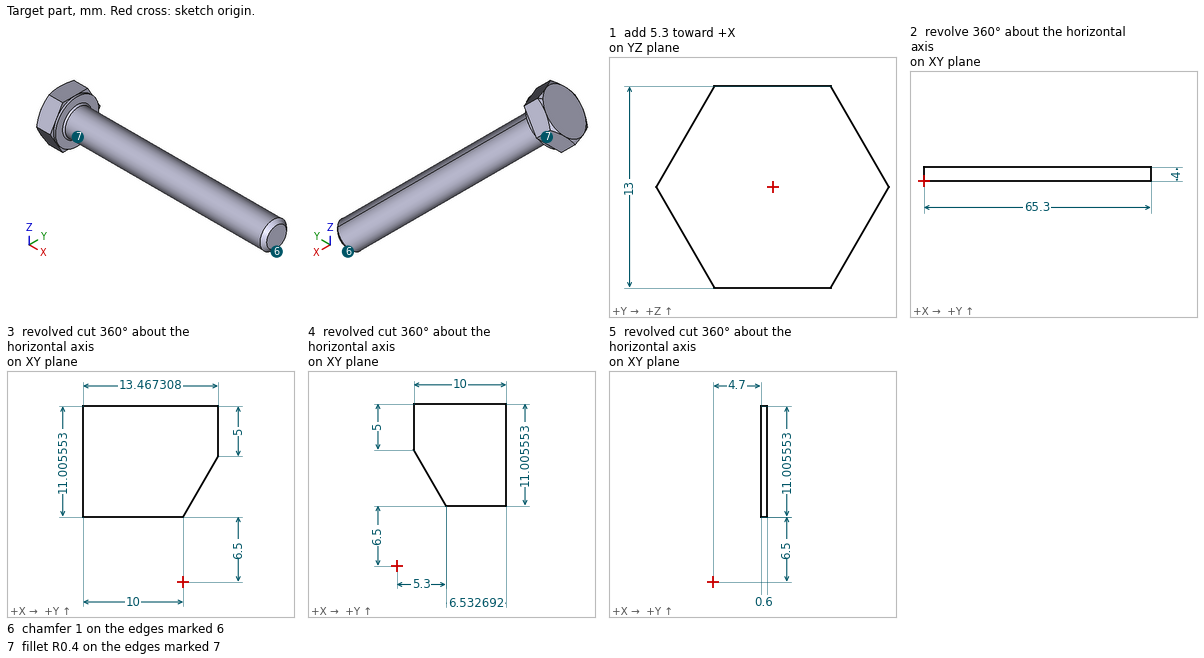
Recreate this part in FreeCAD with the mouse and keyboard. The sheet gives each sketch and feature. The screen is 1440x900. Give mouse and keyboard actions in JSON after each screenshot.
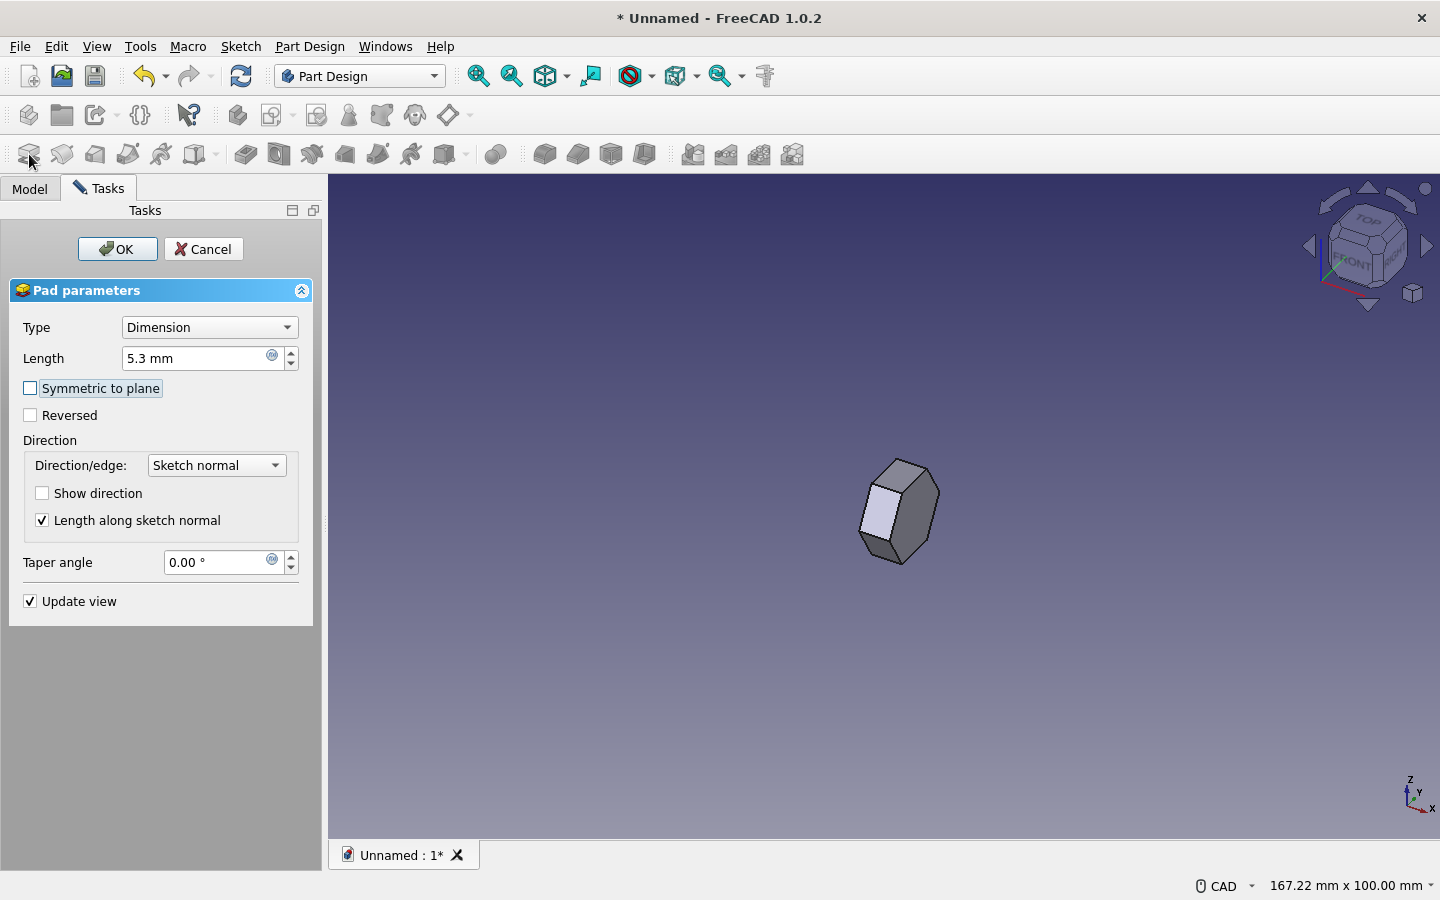
{"action": "left_click", "coordinate": [118, 249]}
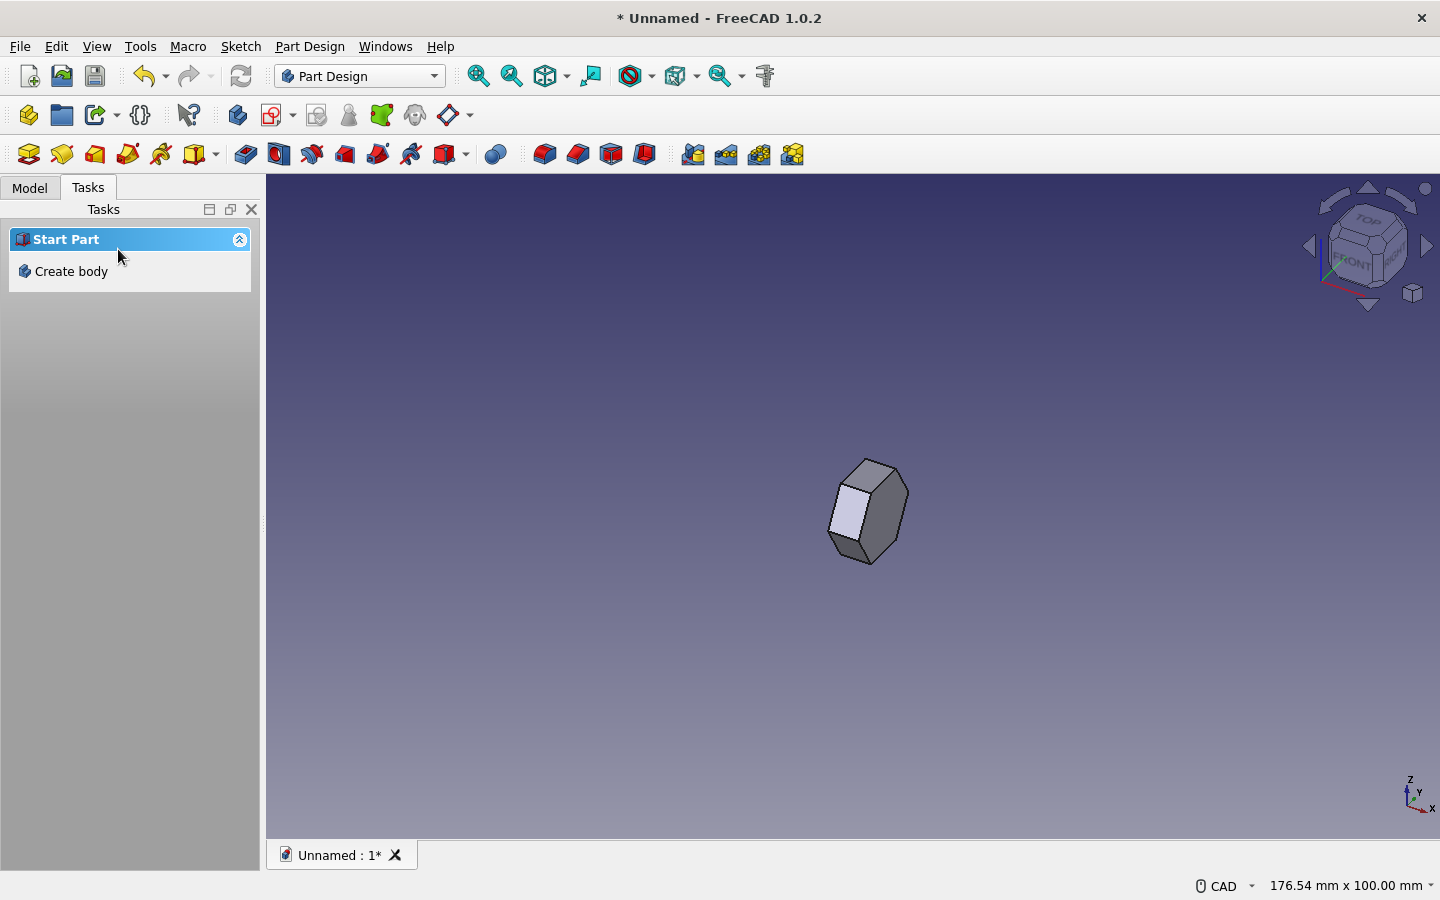
{"action": "left_click", "coordinate": [479, 76]}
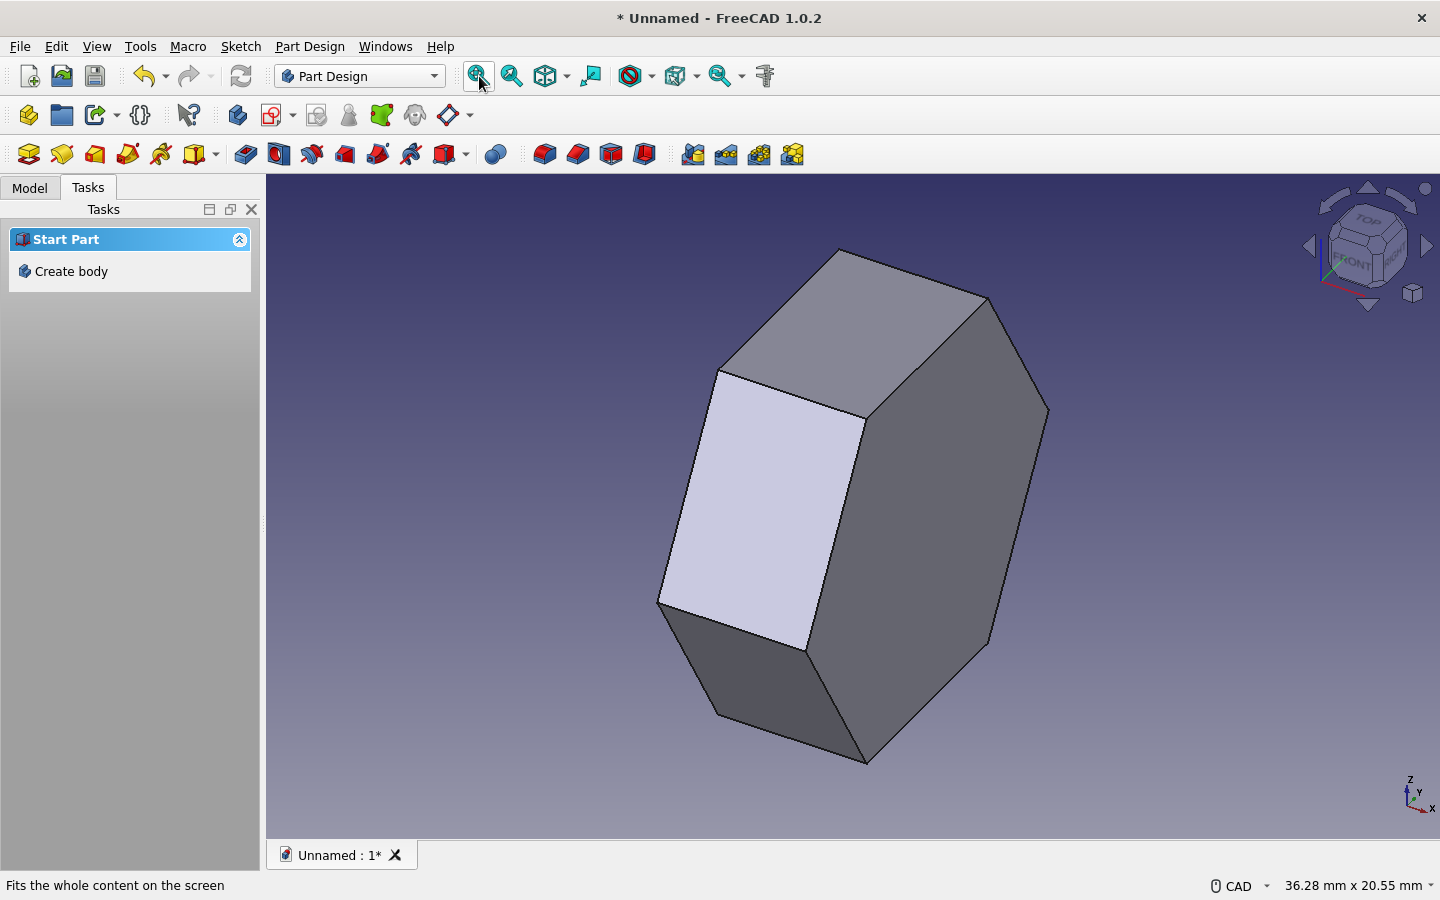
{"action": "left_click", "coordinate": [270, 116]}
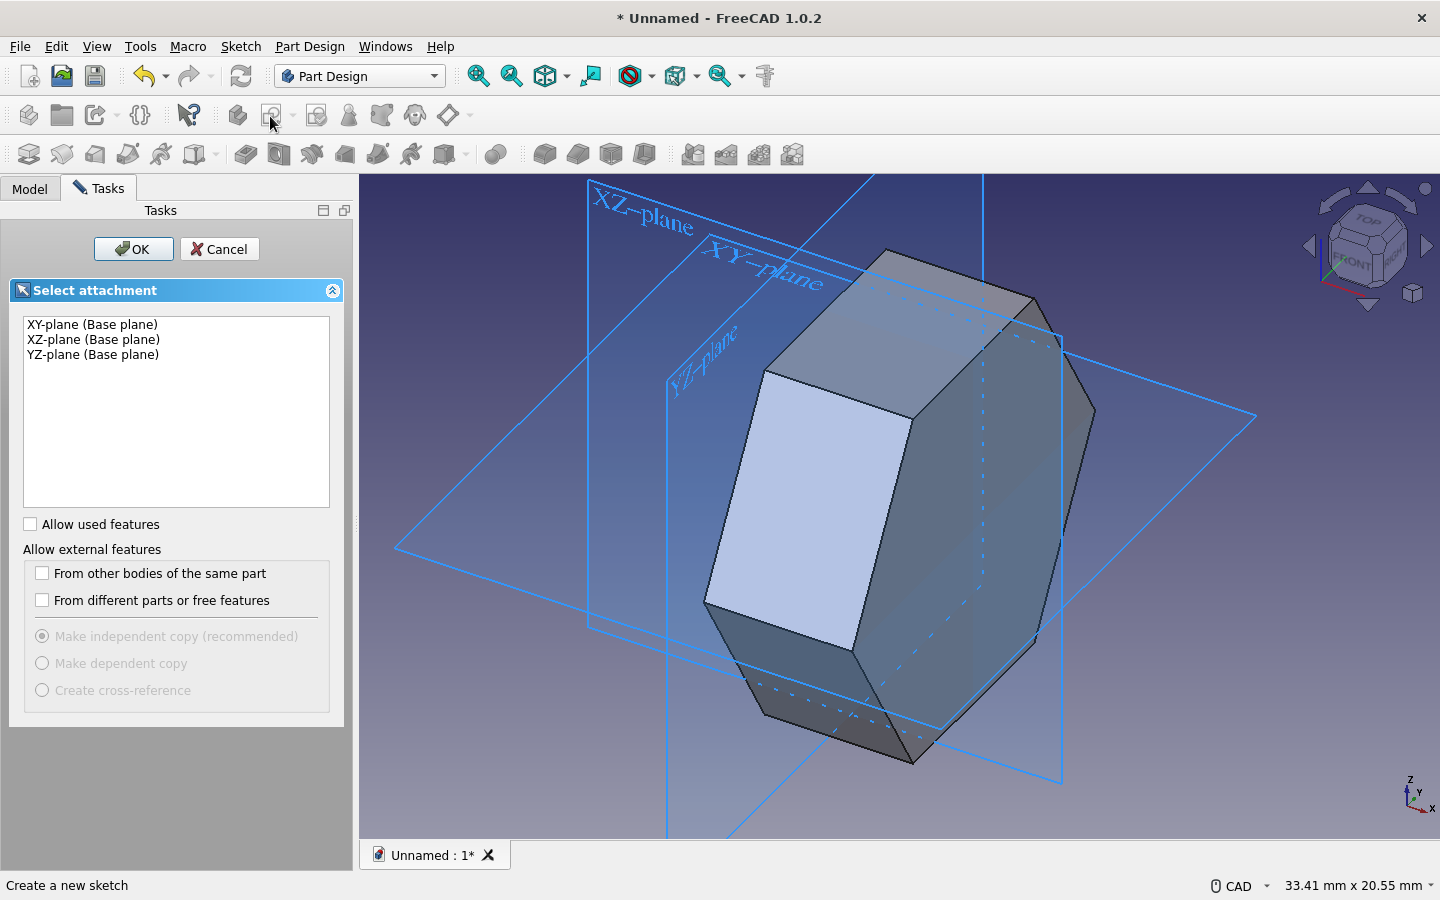
{"action": "left_click", "coordinate": [84, 324]}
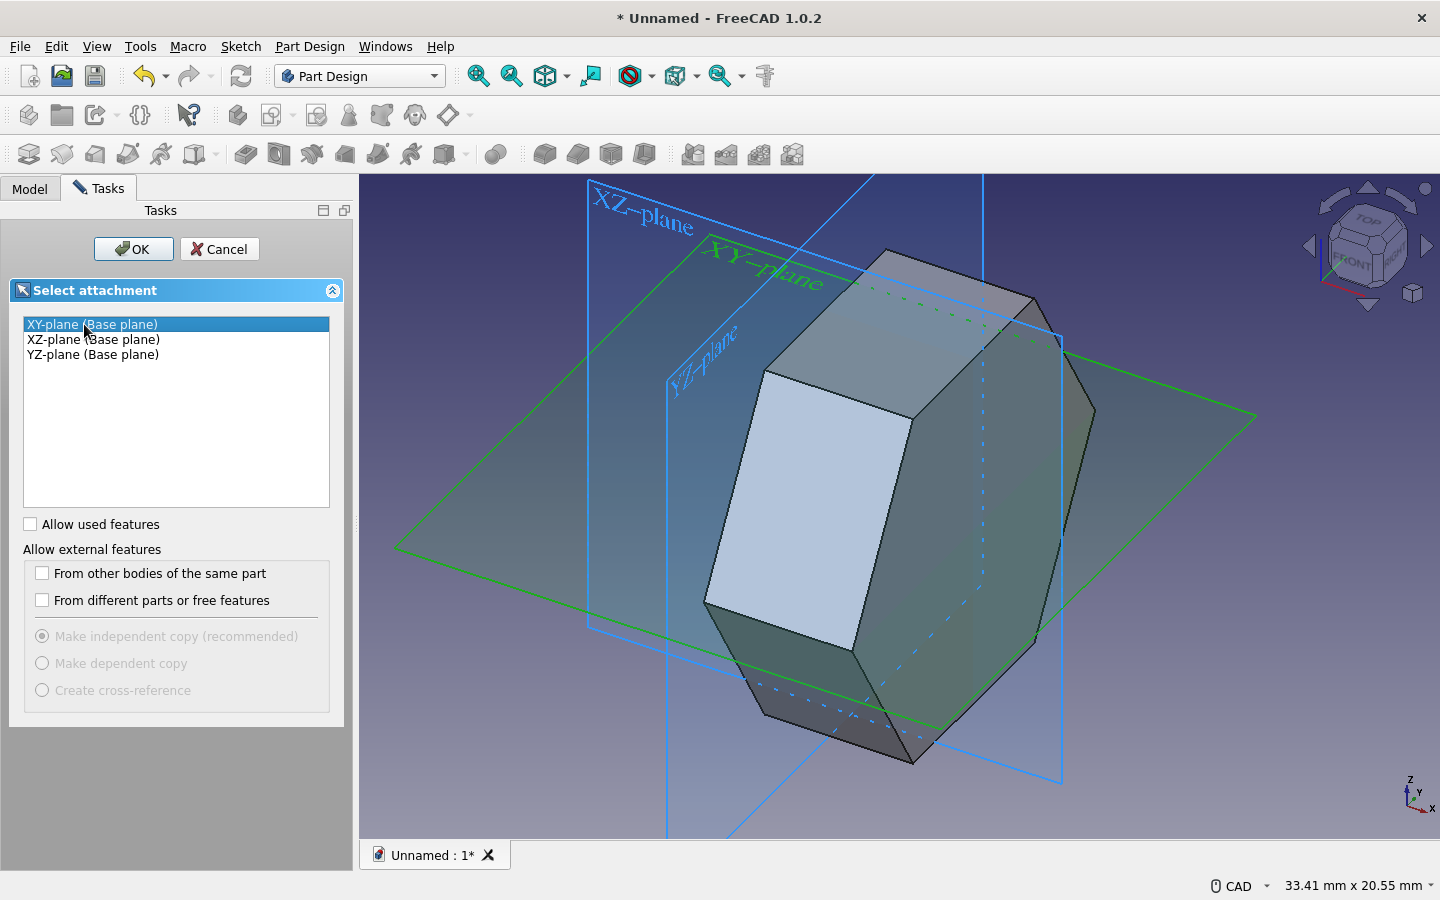
{"action": "left_click", "coordinate": [134, 249]}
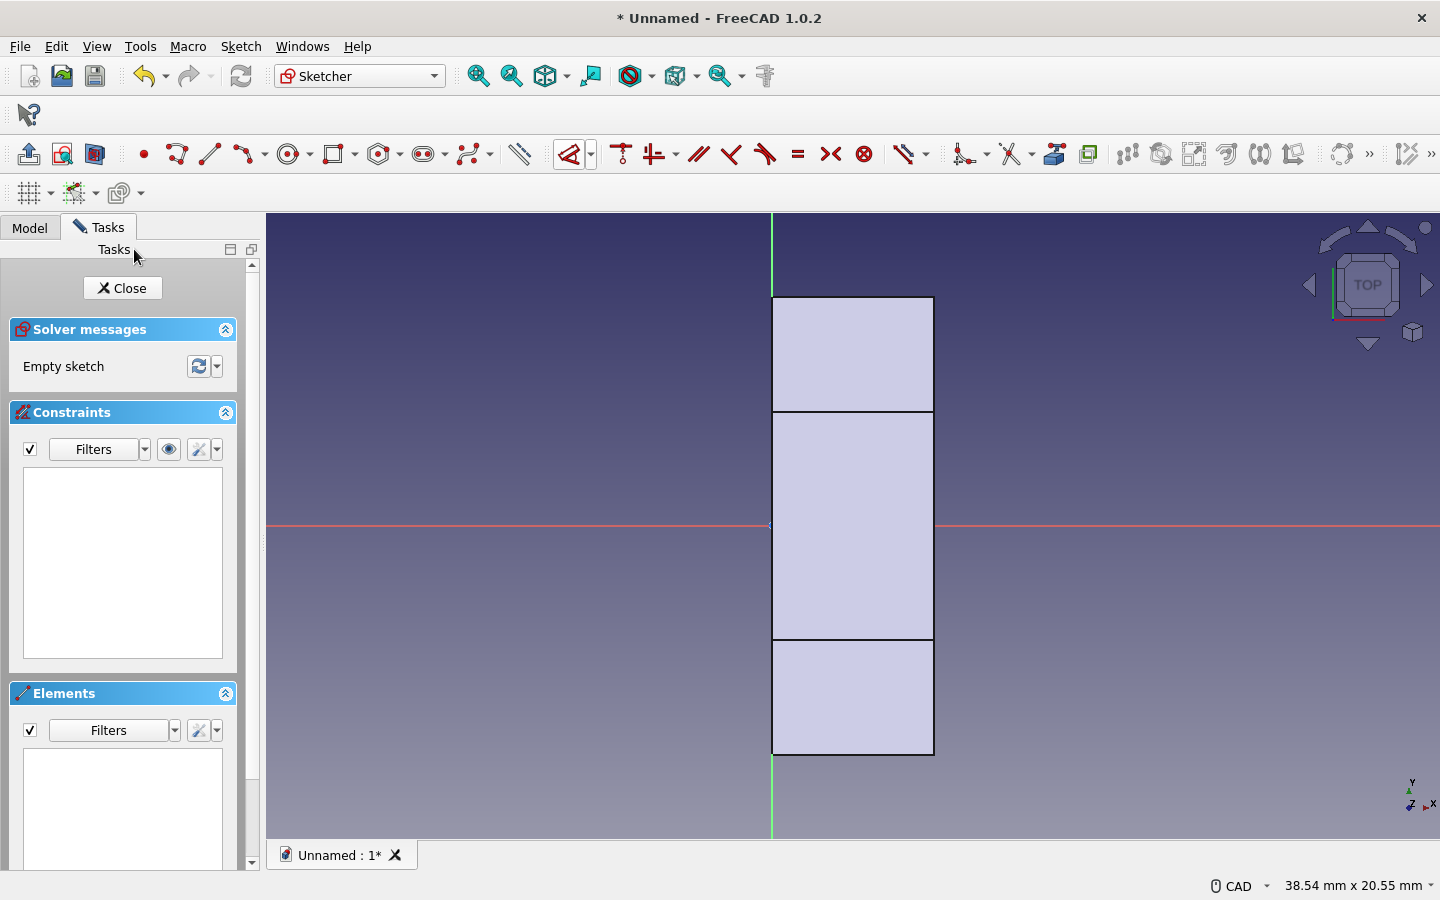
{"action": "left_click", "coordinate": [95, 154]}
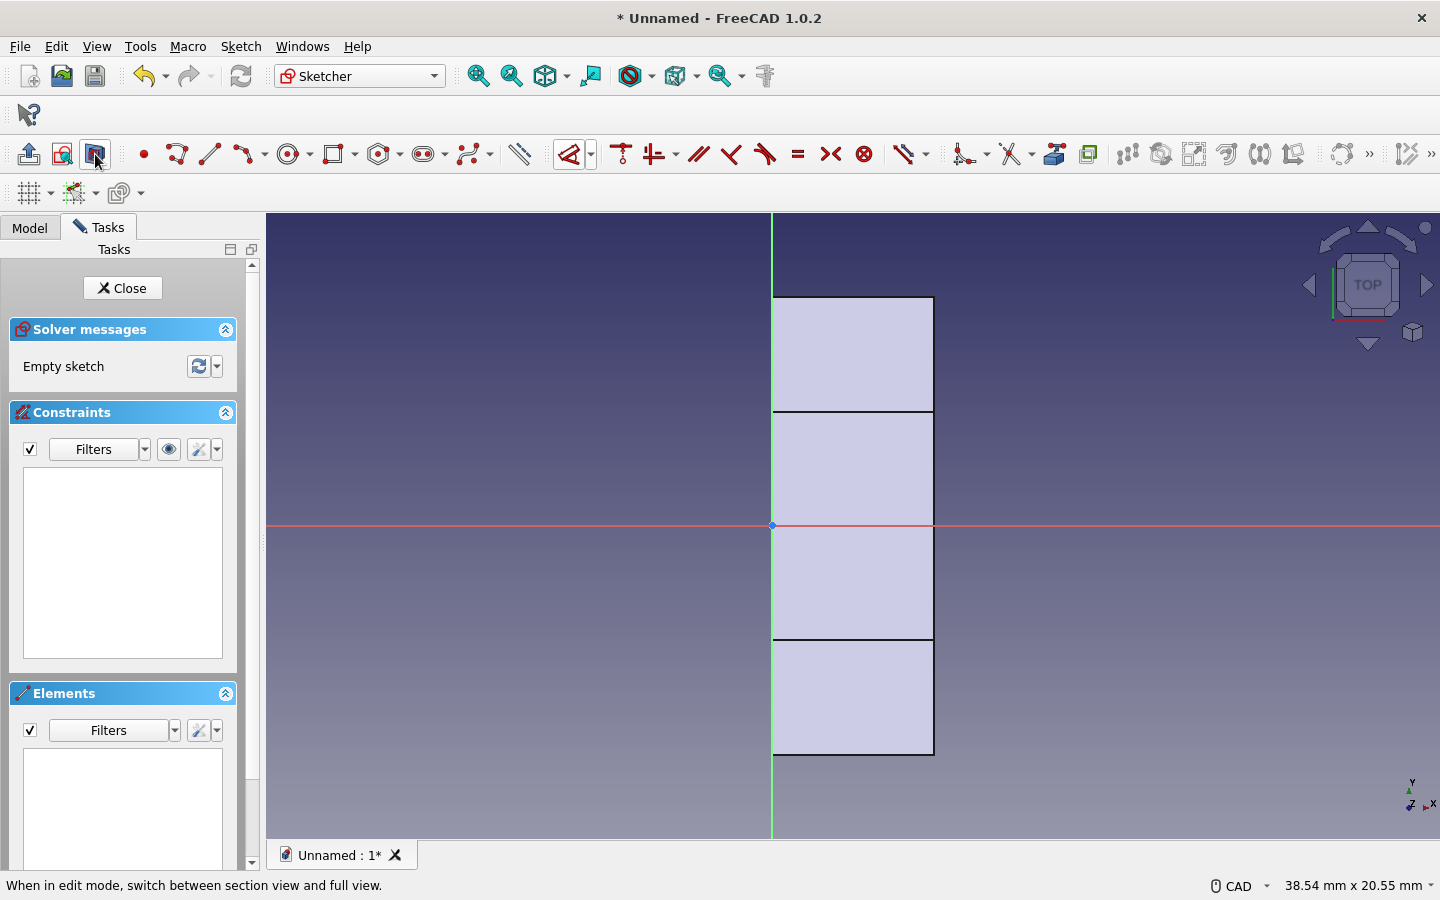
{"action": "scroll", "coordinate": [294, 561], "scroll_direction": "down", "scroll_amount": 5}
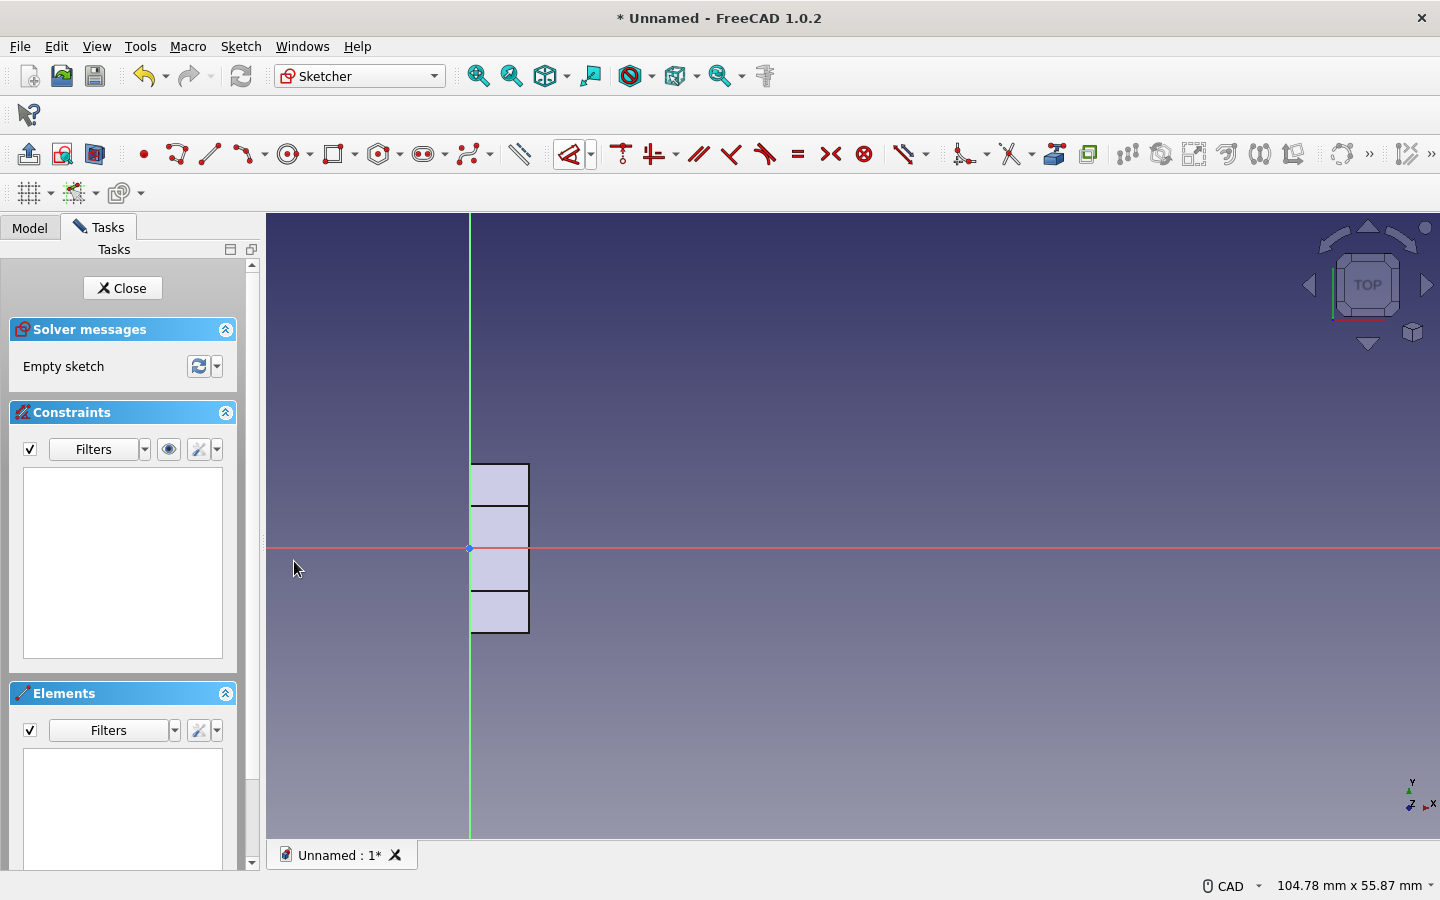
{"action": "left_click", "coordinate": [332, 154]}